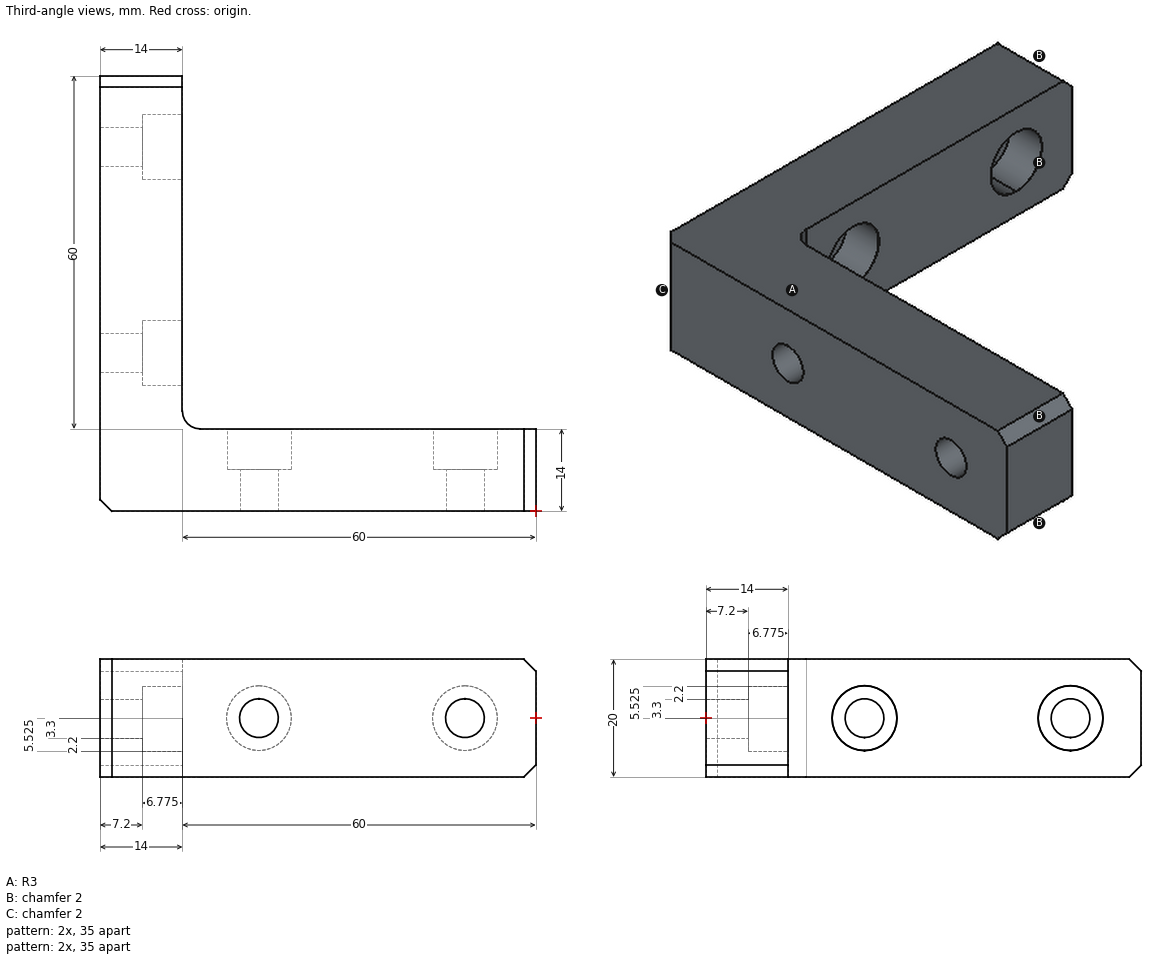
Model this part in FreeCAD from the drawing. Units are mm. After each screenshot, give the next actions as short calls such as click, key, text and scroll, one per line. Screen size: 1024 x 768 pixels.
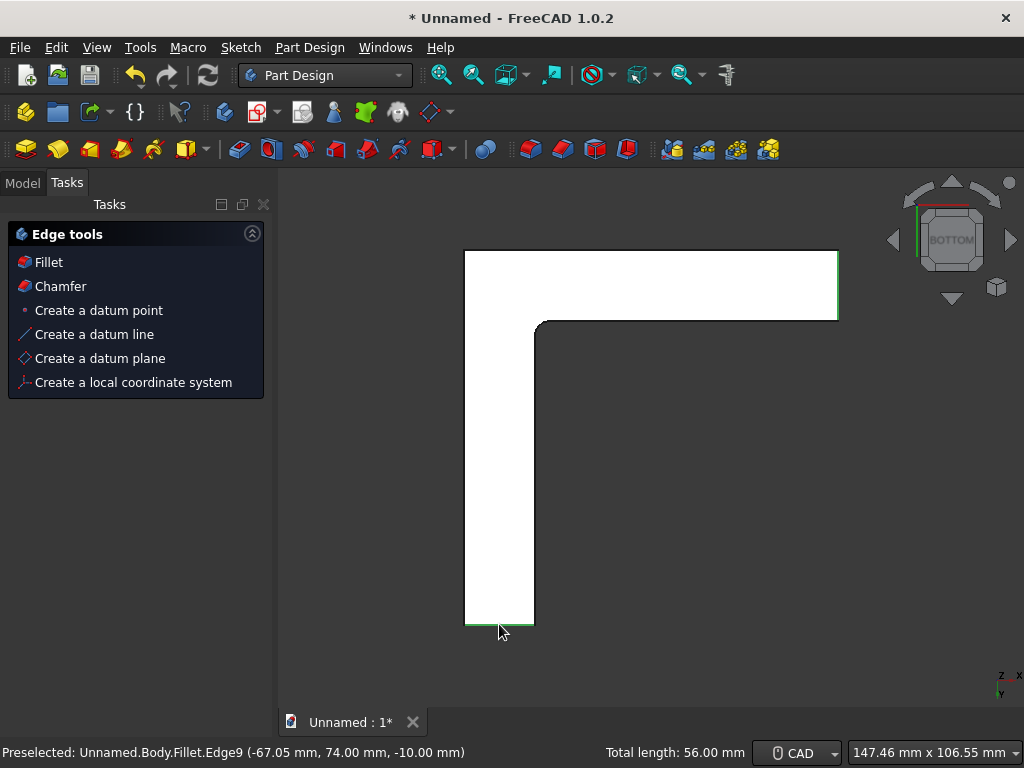
click(564, 150)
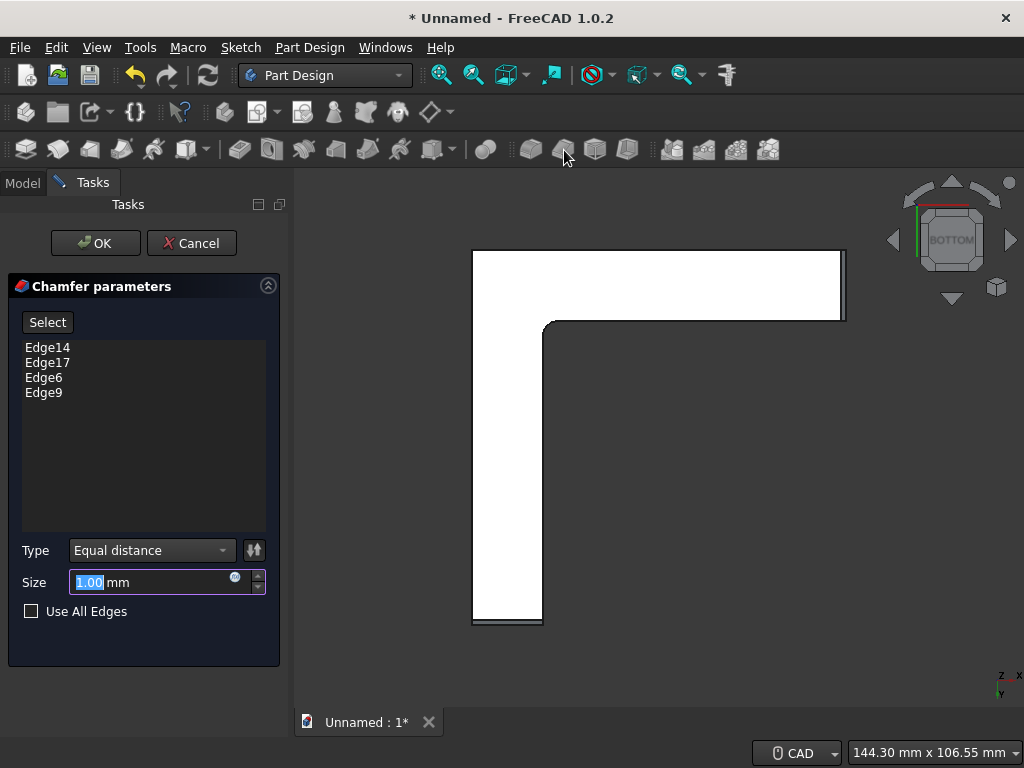
text(2)
key(Tab)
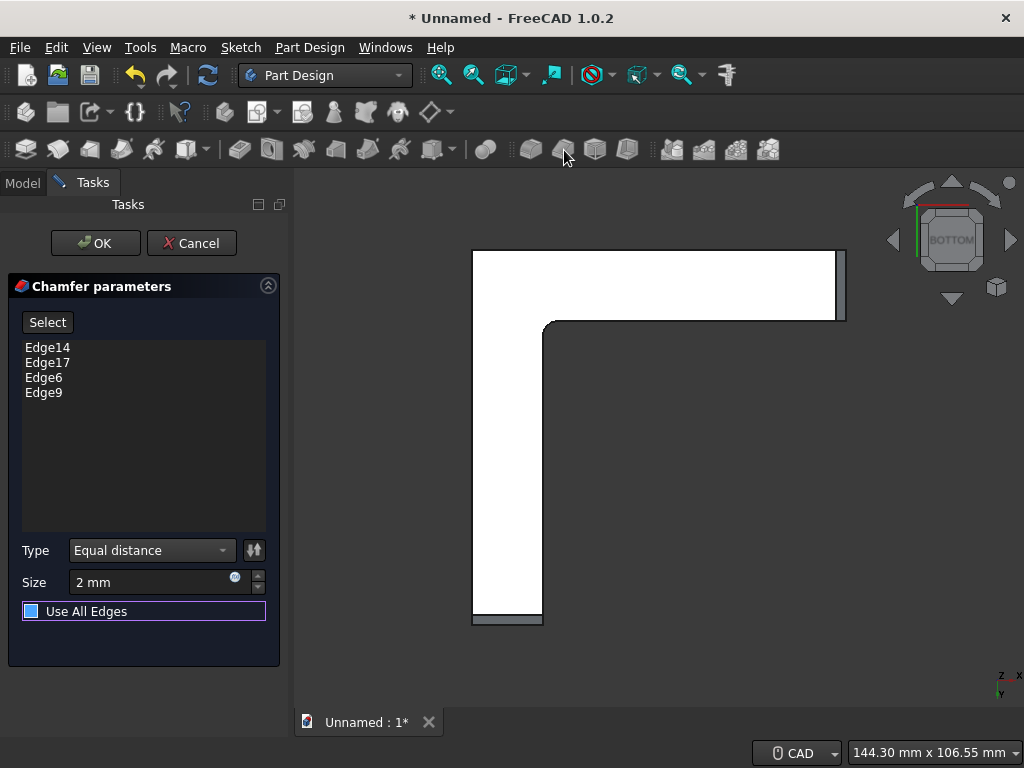
click(96, 243)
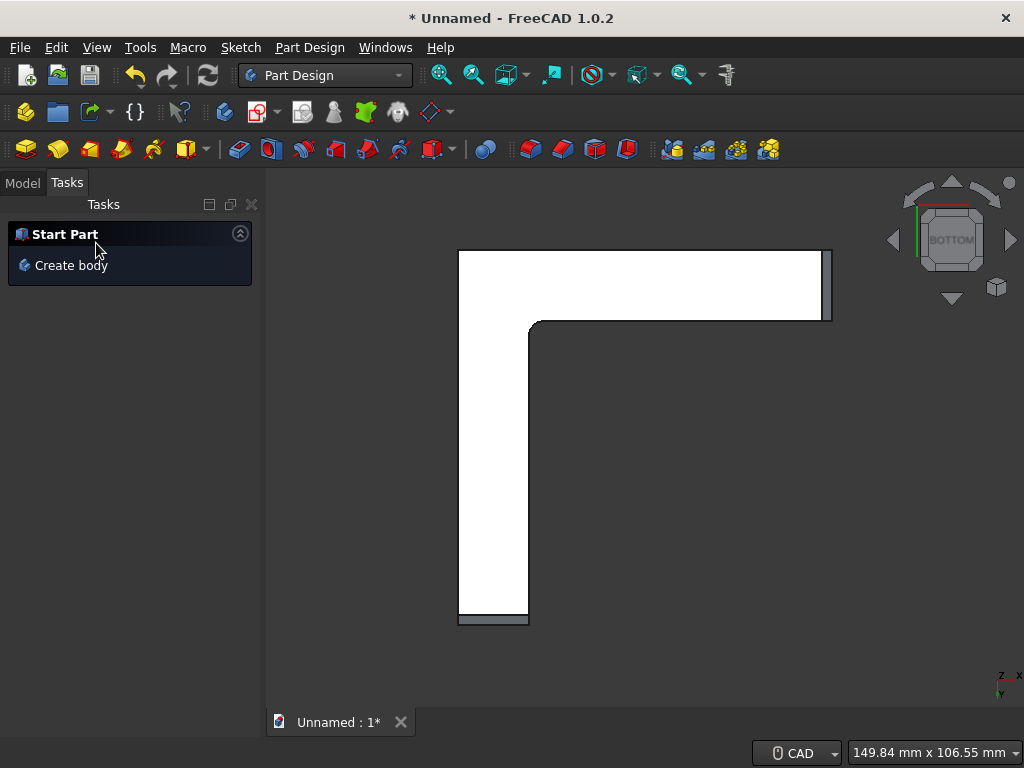
key(0)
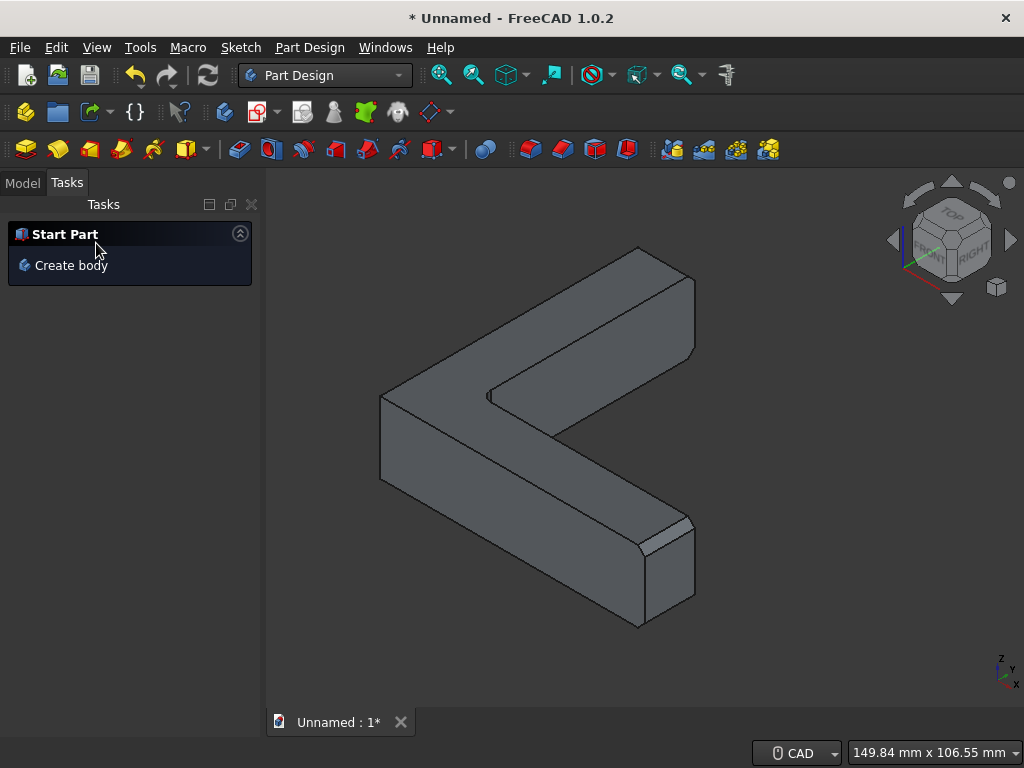
key(2)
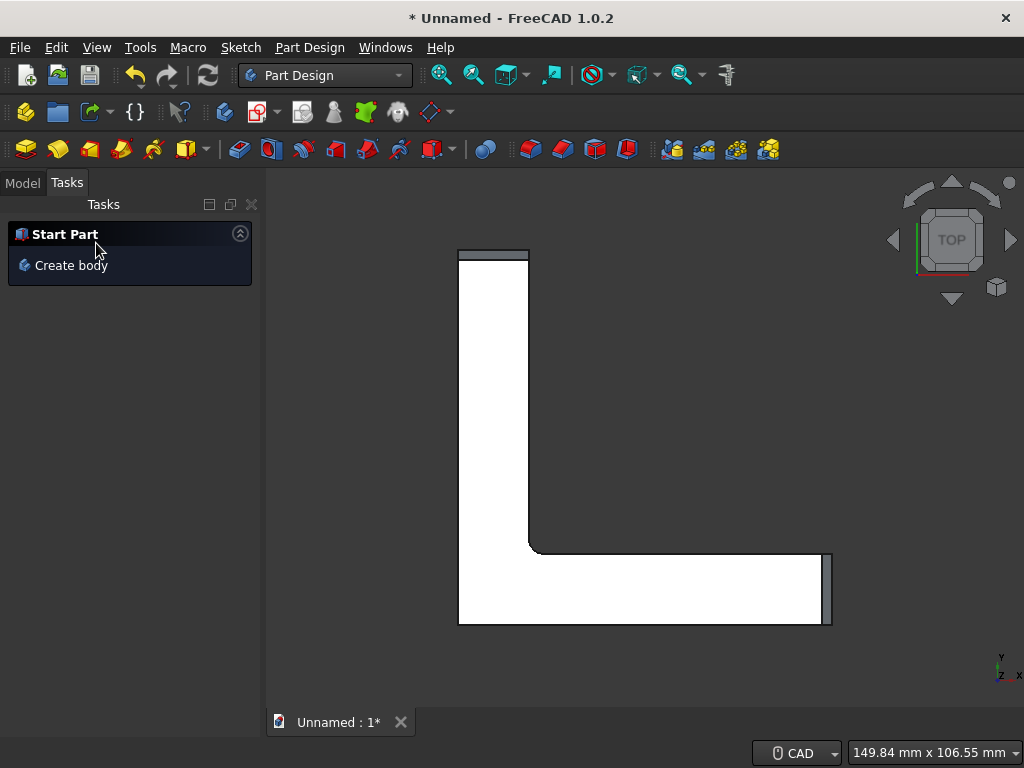
key(1)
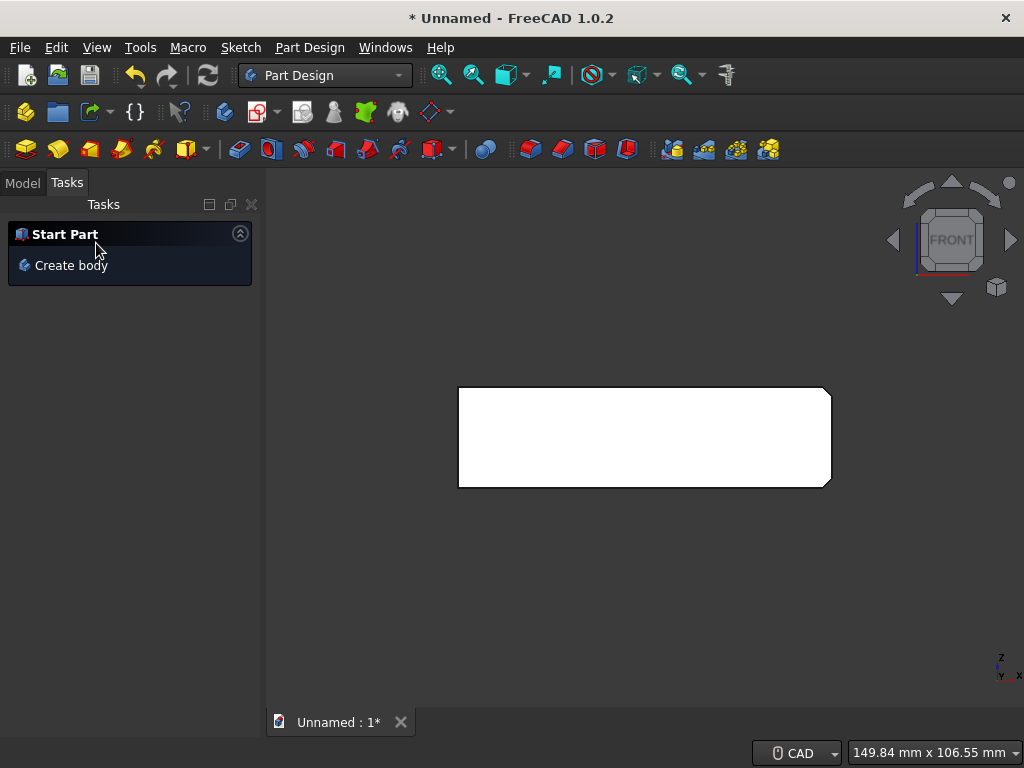
click(458, 437)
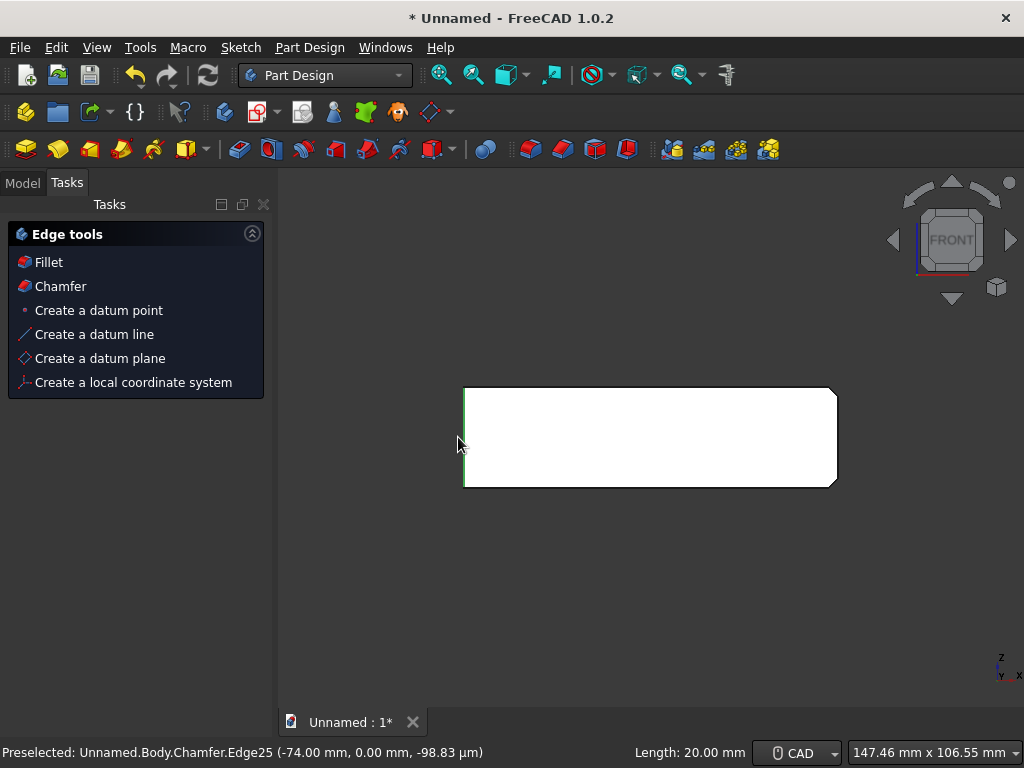
click(564, 150)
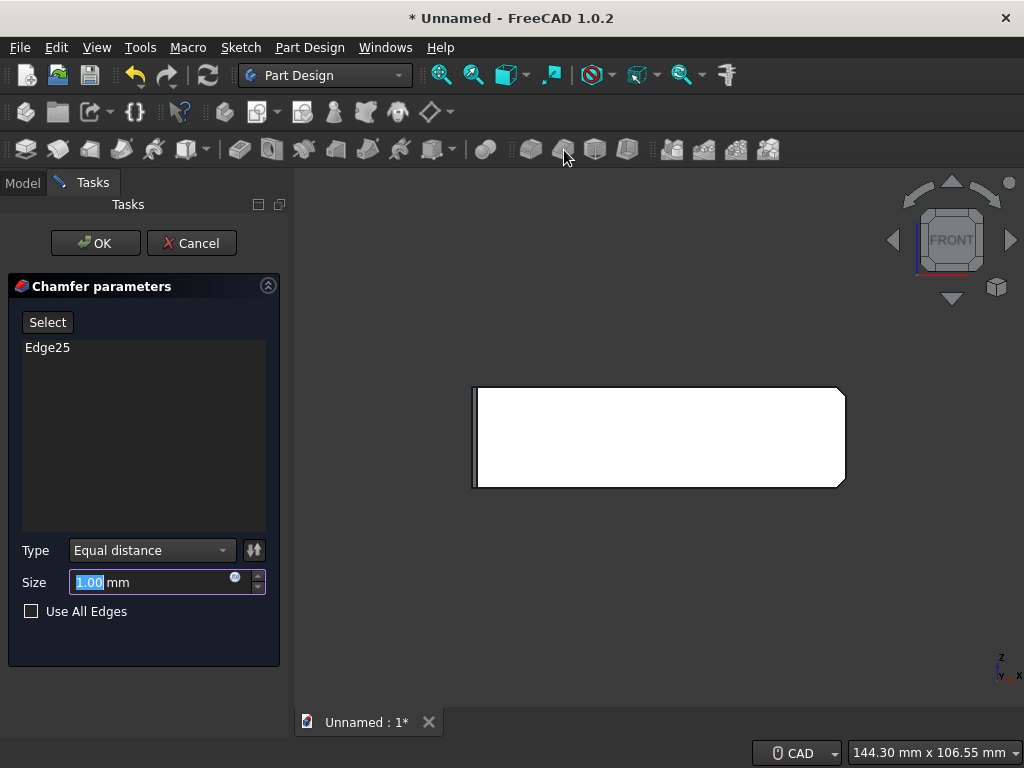
text(2)
key(Tab)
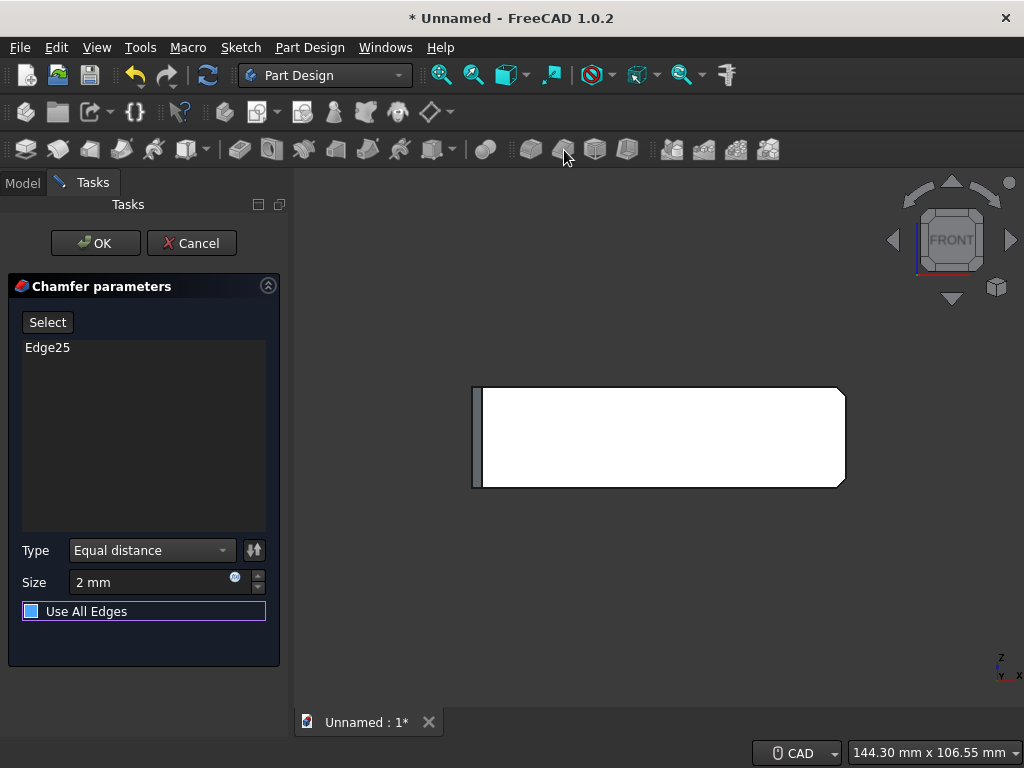
click(96, 243)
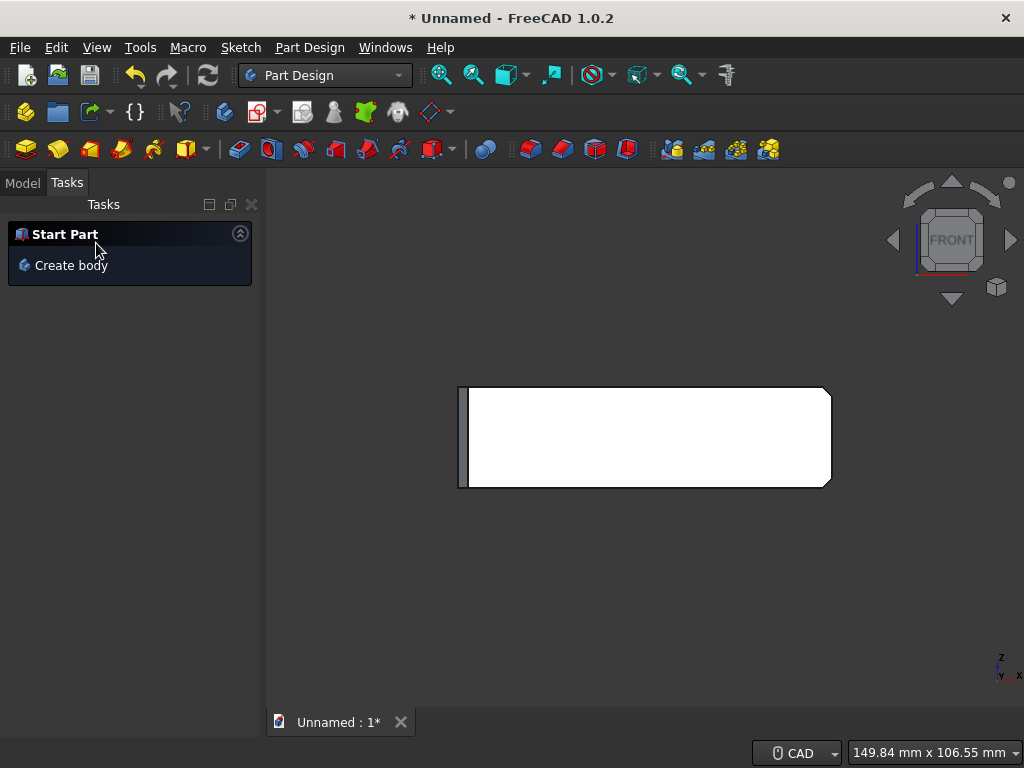
click(23, 182)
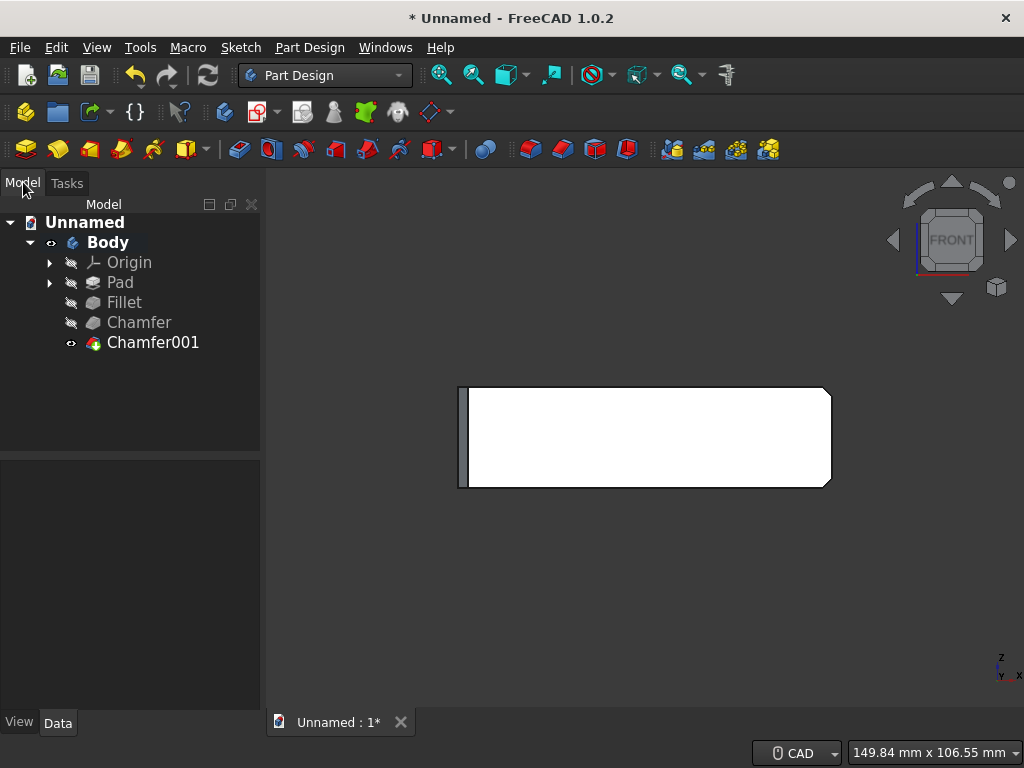
click(50, 263)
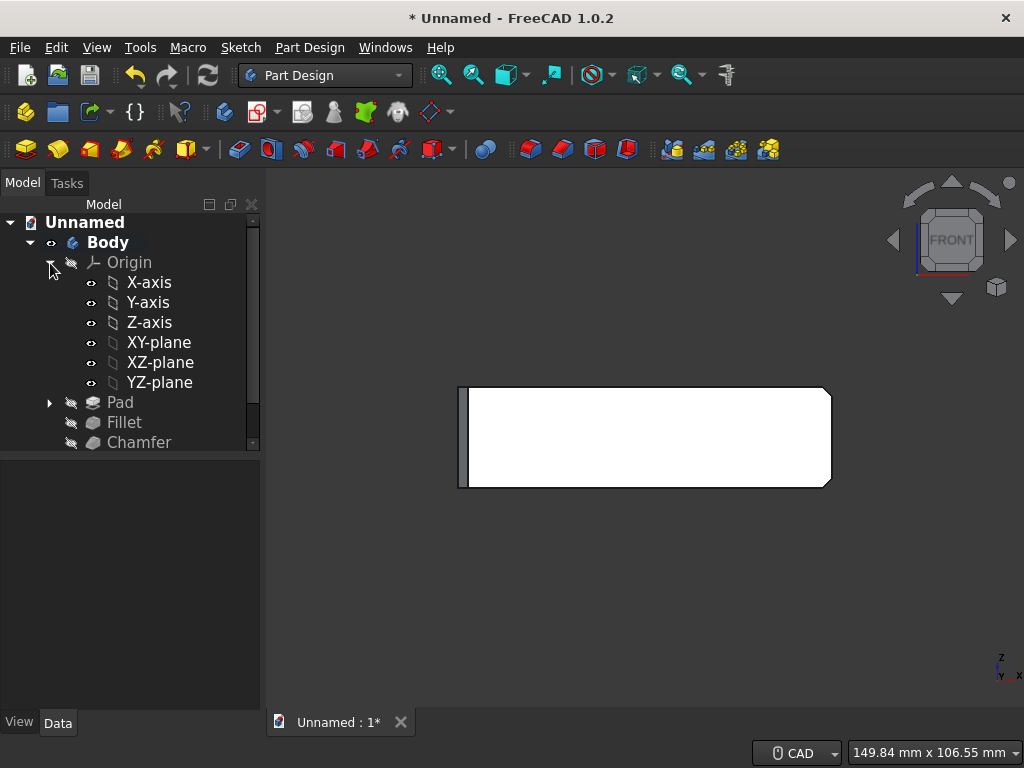
click(136, 363)